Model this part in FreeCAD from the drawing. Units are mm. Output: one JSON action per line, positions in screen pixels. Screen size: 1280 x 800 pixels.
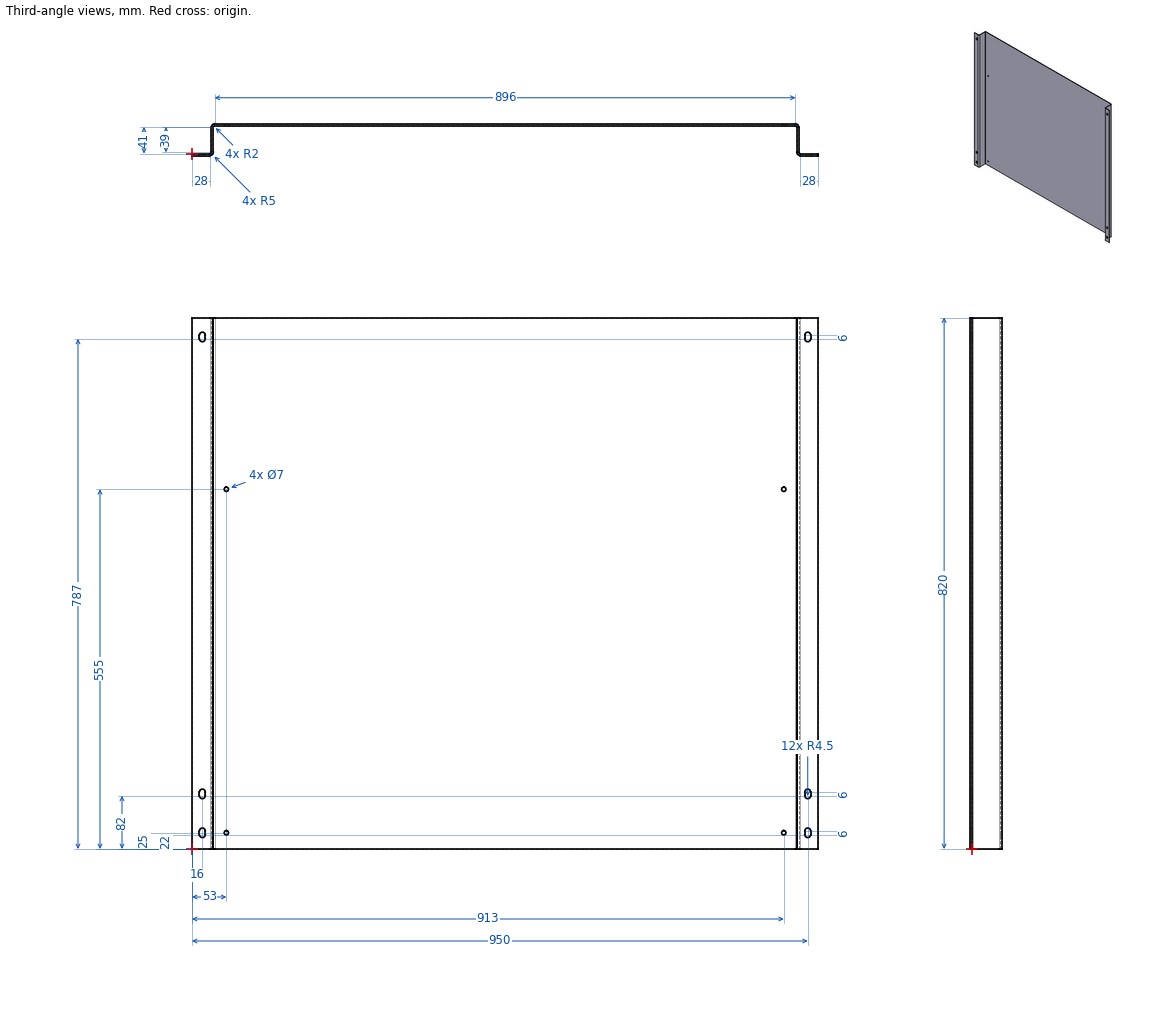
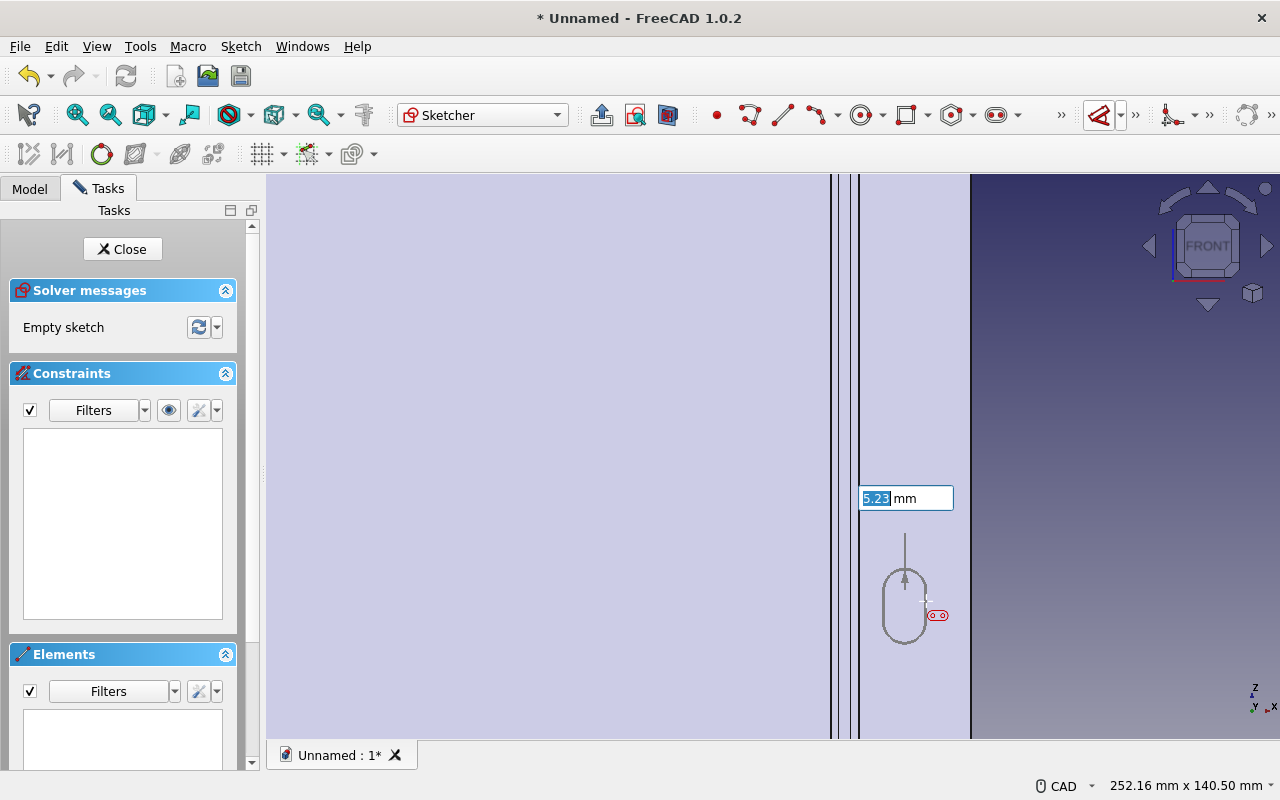
{"action": "left_click", "coordinate": [925, 601]}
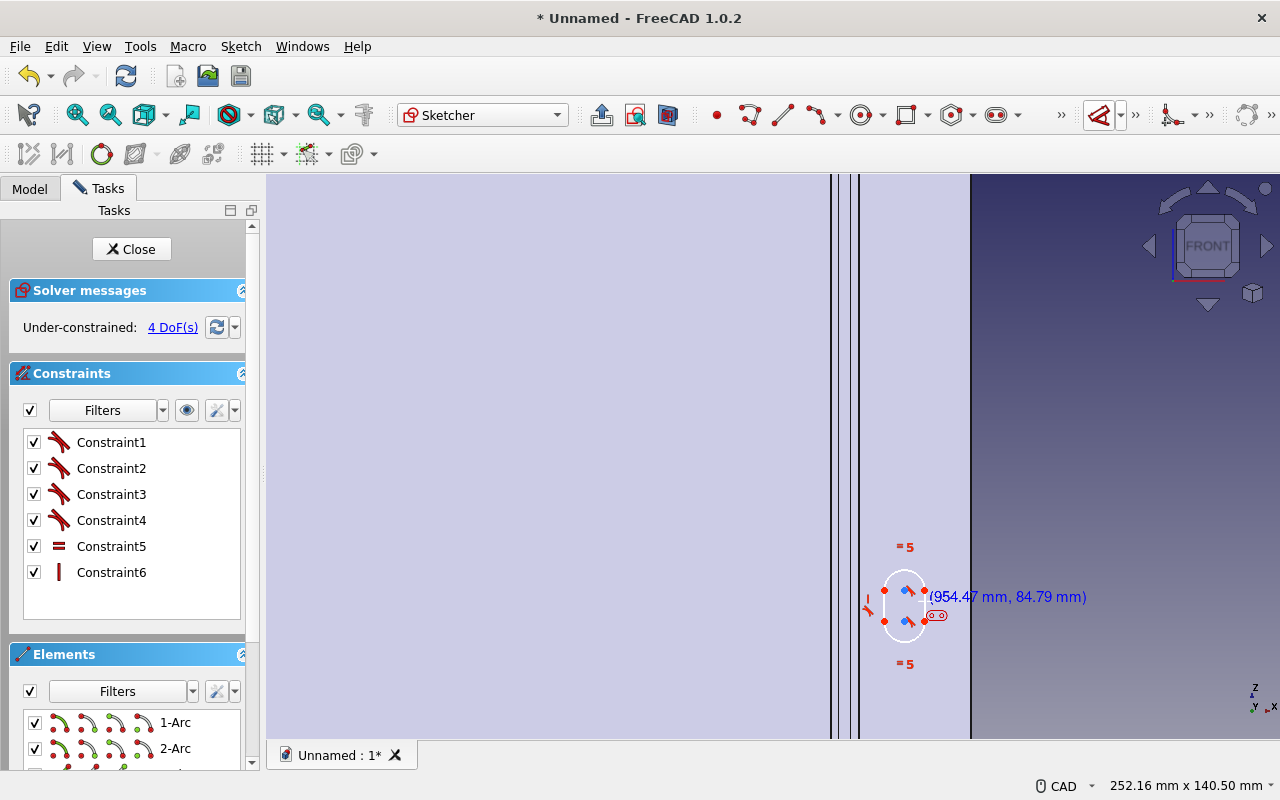
{"action": "scroll", "coordinate": [916, 596], "scroll_direction": "down", "scroll_amount": 11}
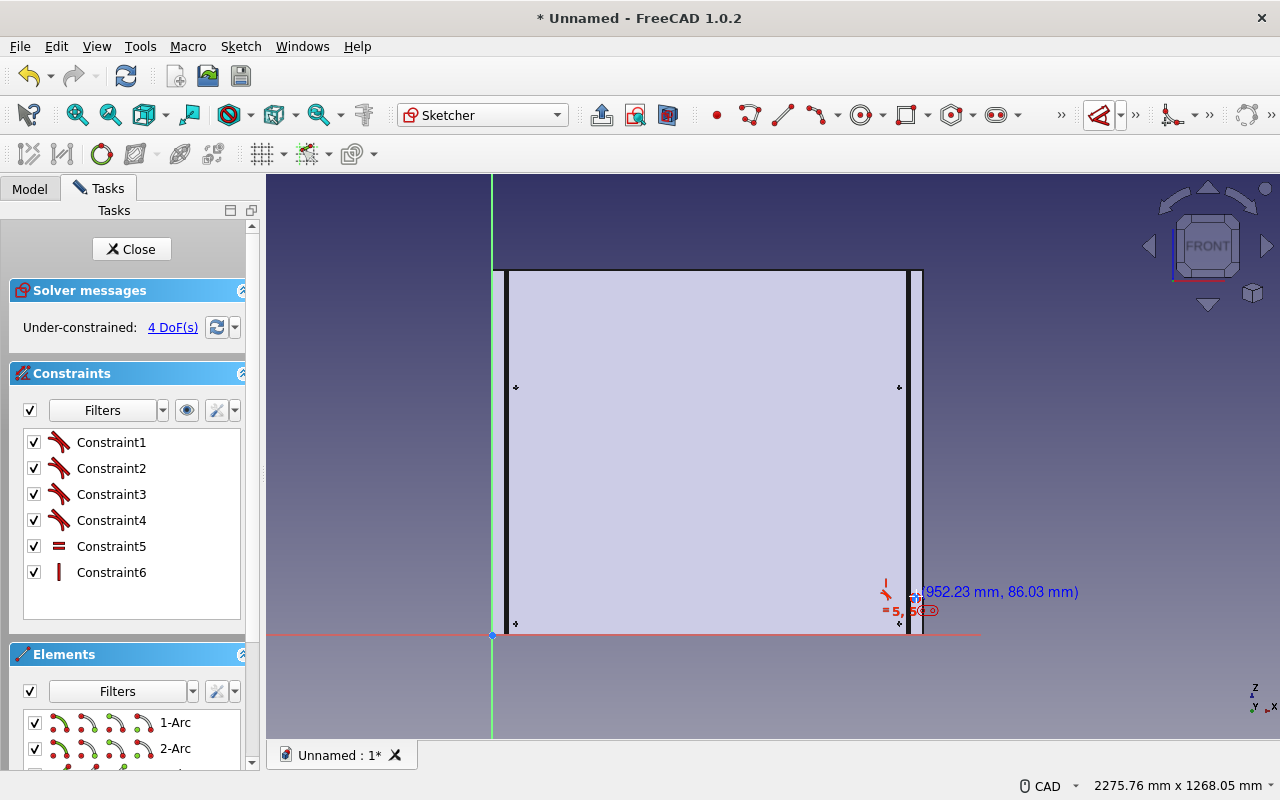
{"action": "scroll", "coordinate": [916, 625], "scroll_direction": "up", "scroll_amount": 13}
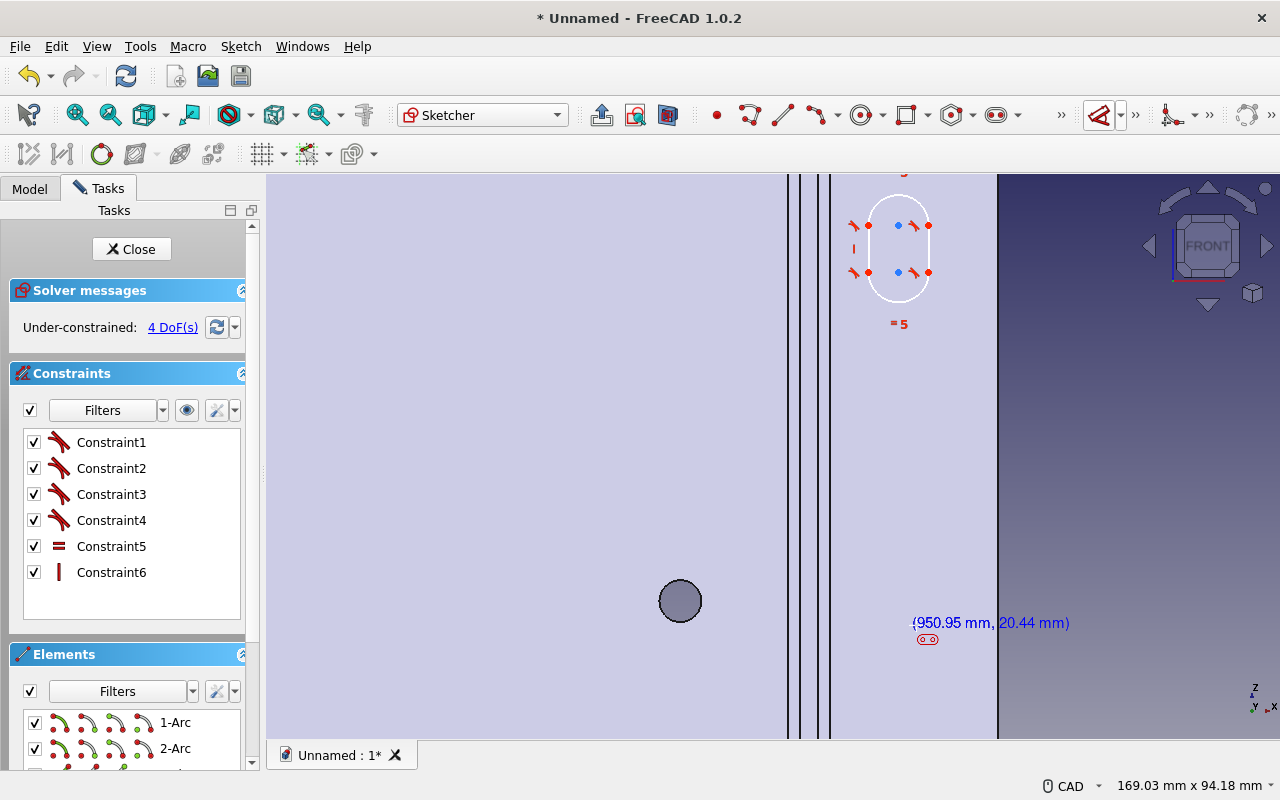
{"action": "scroll", "coordinate": [916, 625], "scroll_direction": "down", "scroll_amount": 13}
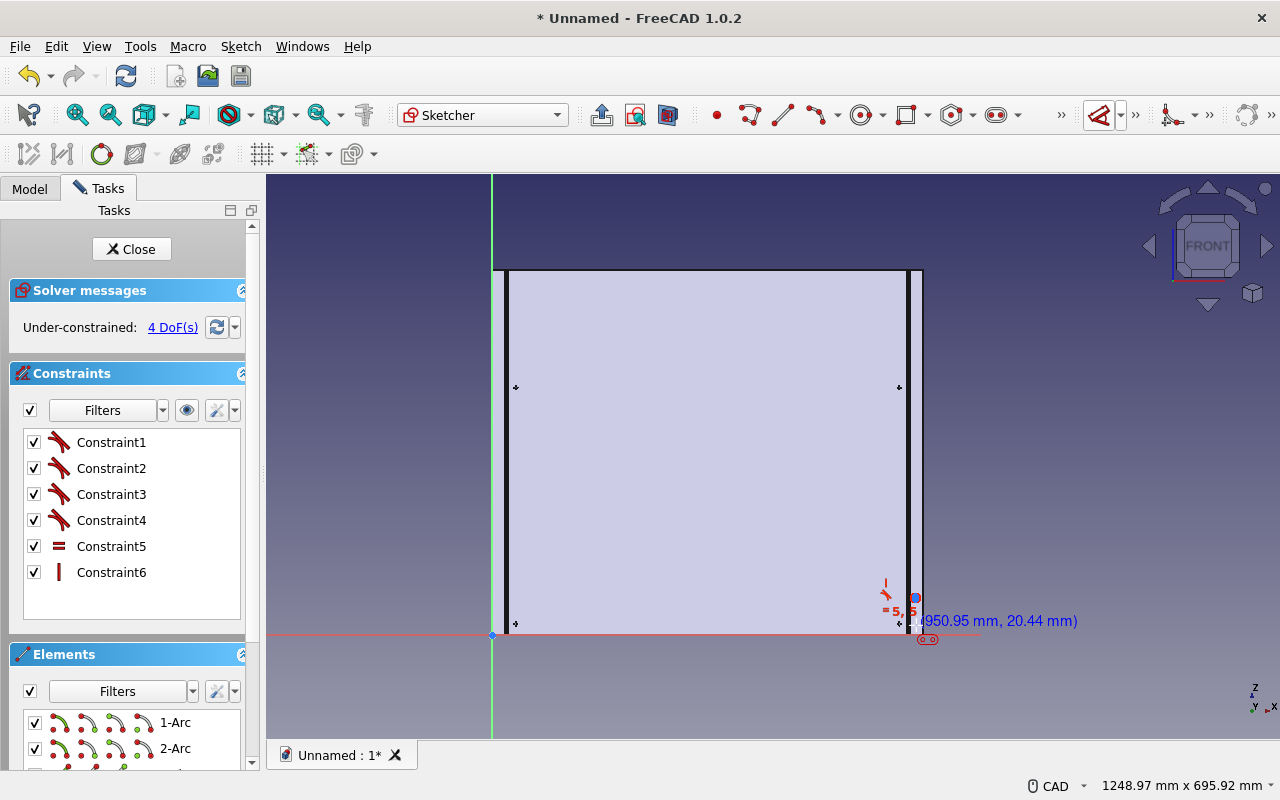
{"action": "scroll", "coordinate": [916, 625], "scroll_direction": "up", "scroll_amount": 3}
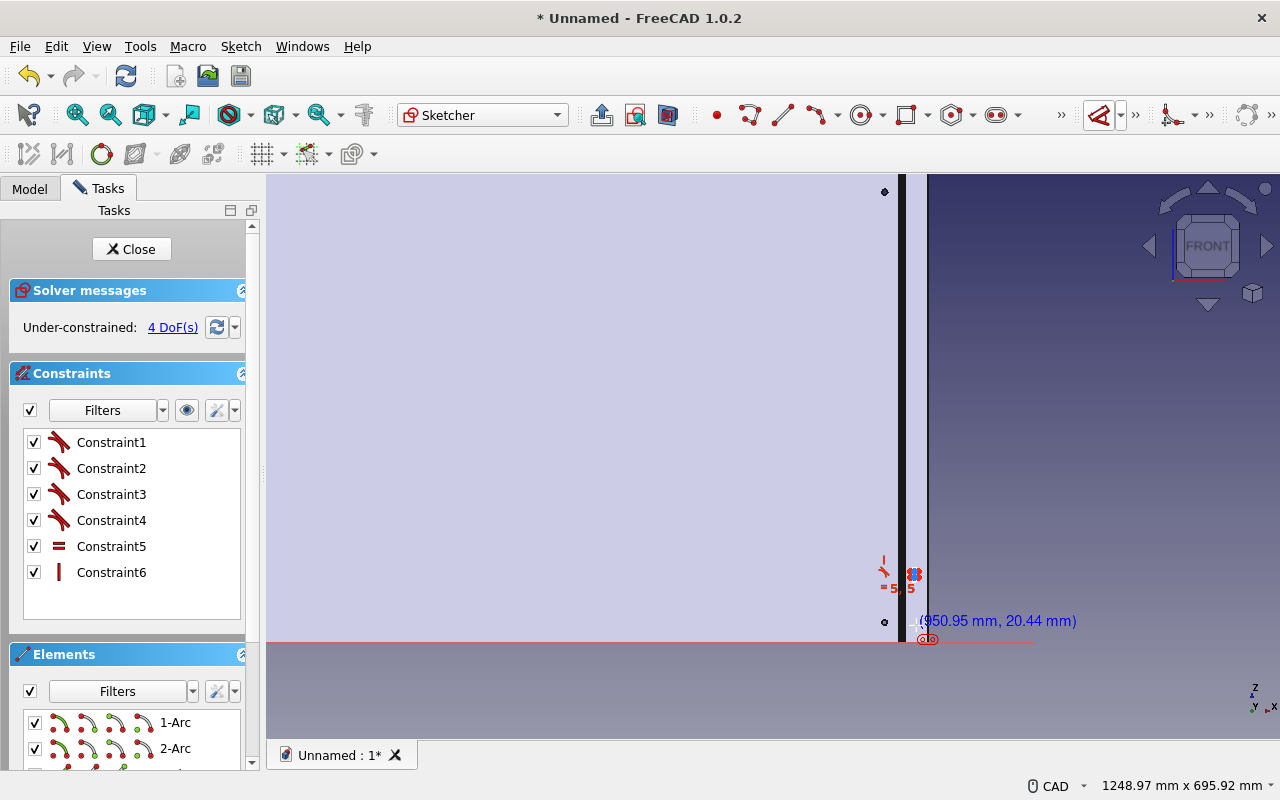
{"action": "left_click", "coordinate": [915, 625]}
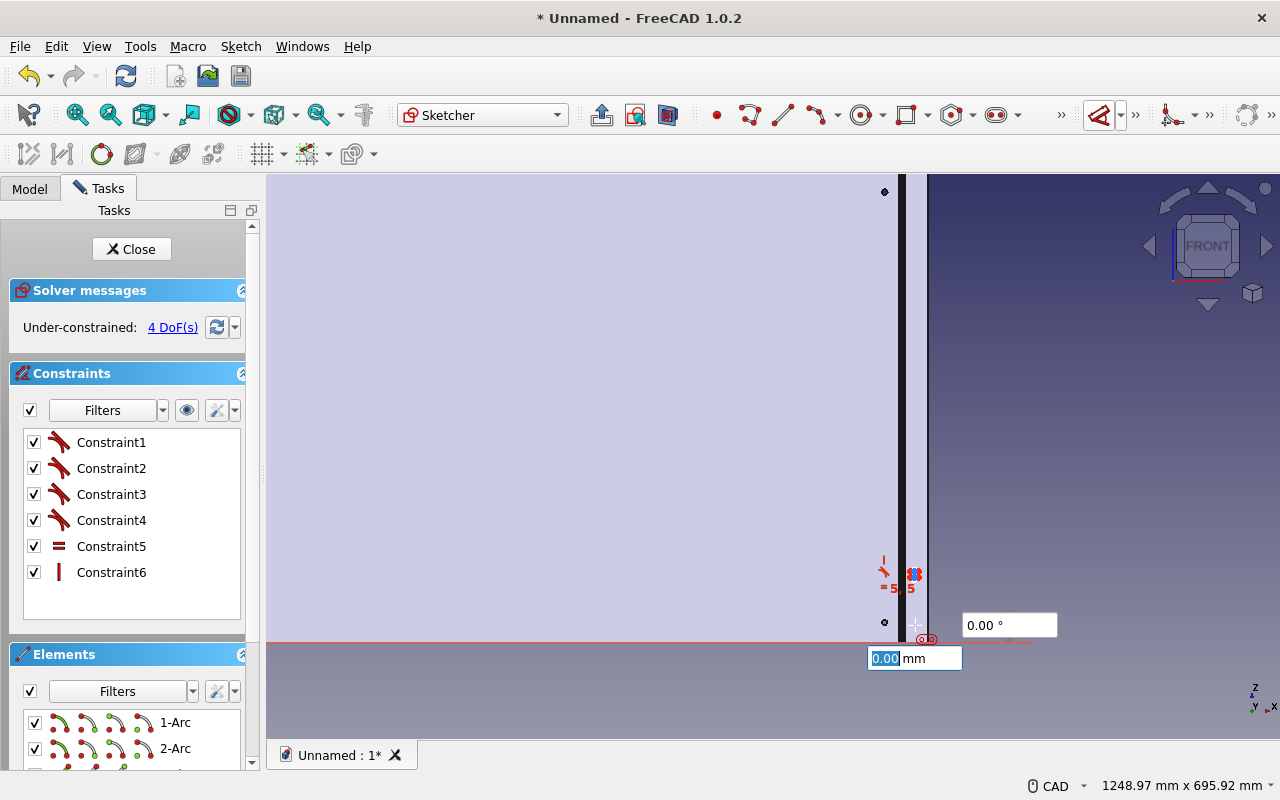
{"action": "scroll", "coordinate": [915, 620], "scroll_direction": "up", "scroll_amount": 6}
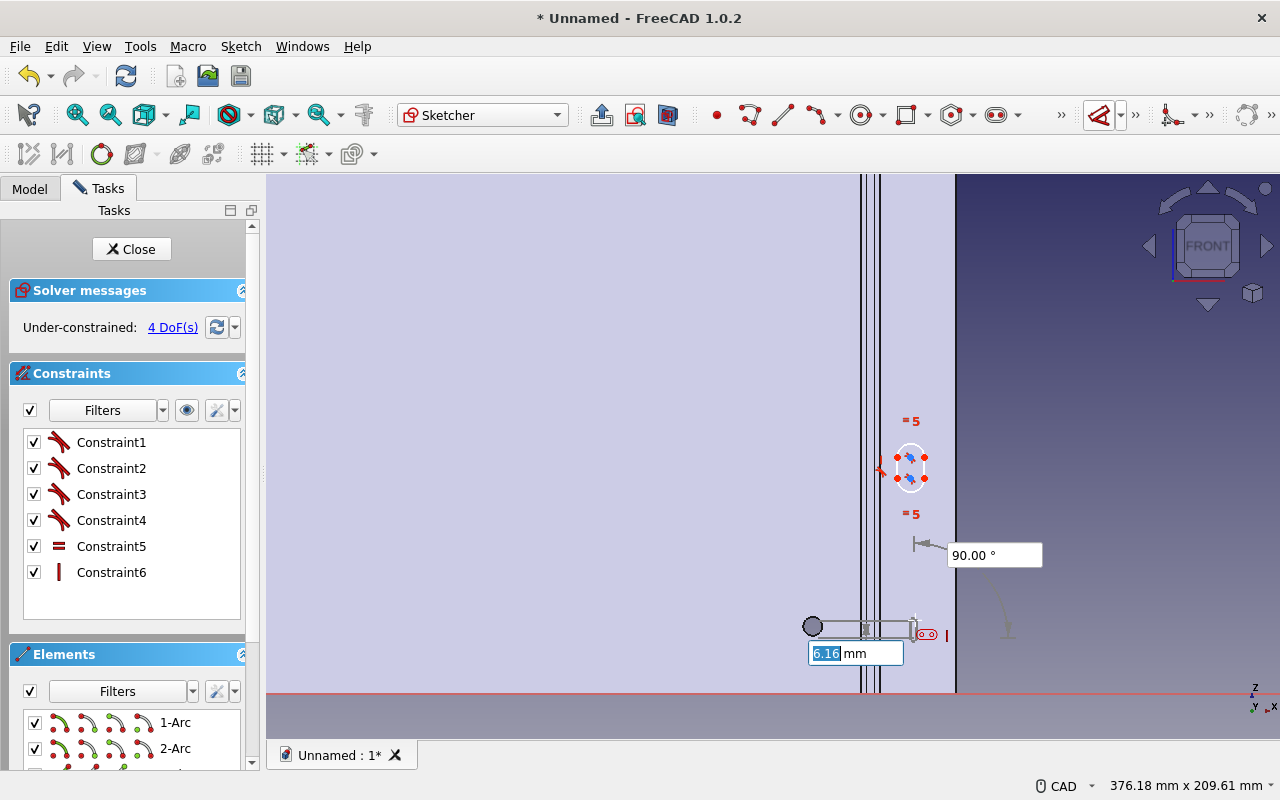
{"action": "left_click", "coordinate": [914, 618]}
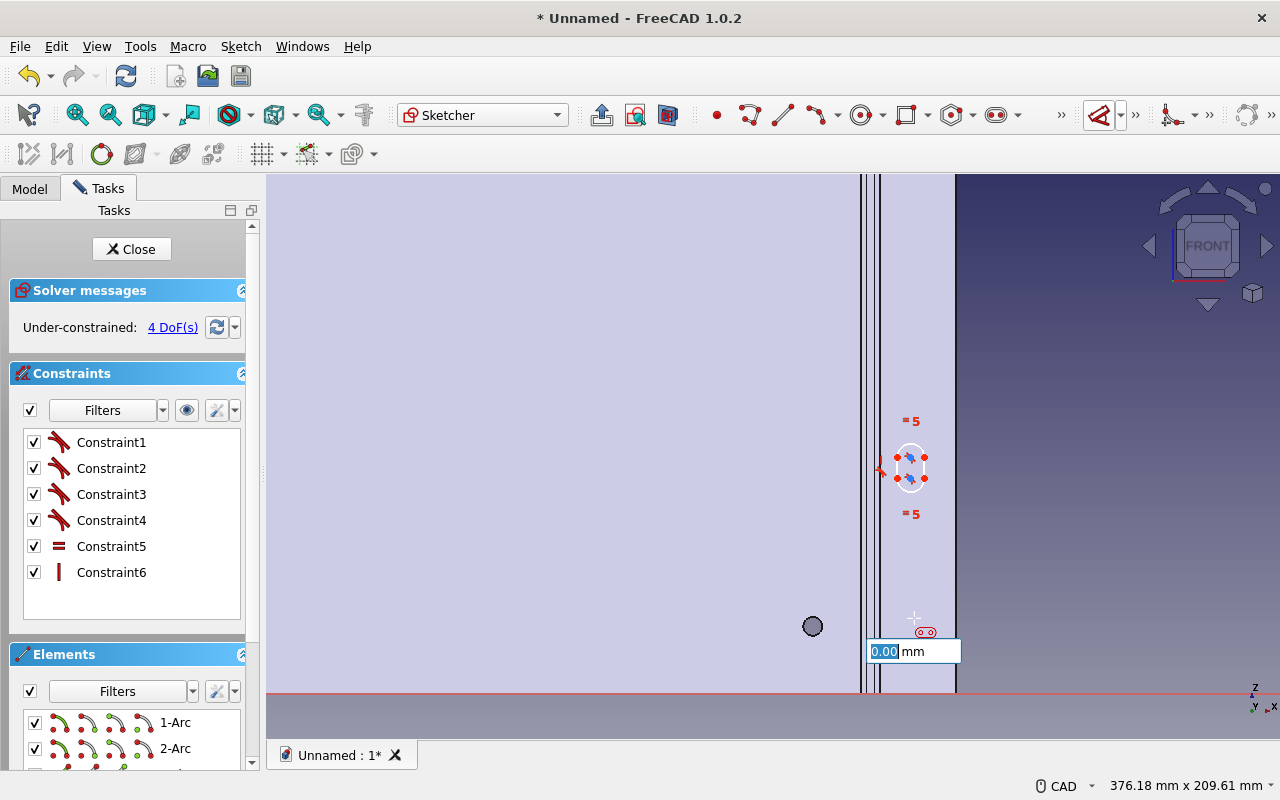
{"action": "scroll", "coordinate": [925, 626], "scroll_direction": "up", "scroll_amount": 2}